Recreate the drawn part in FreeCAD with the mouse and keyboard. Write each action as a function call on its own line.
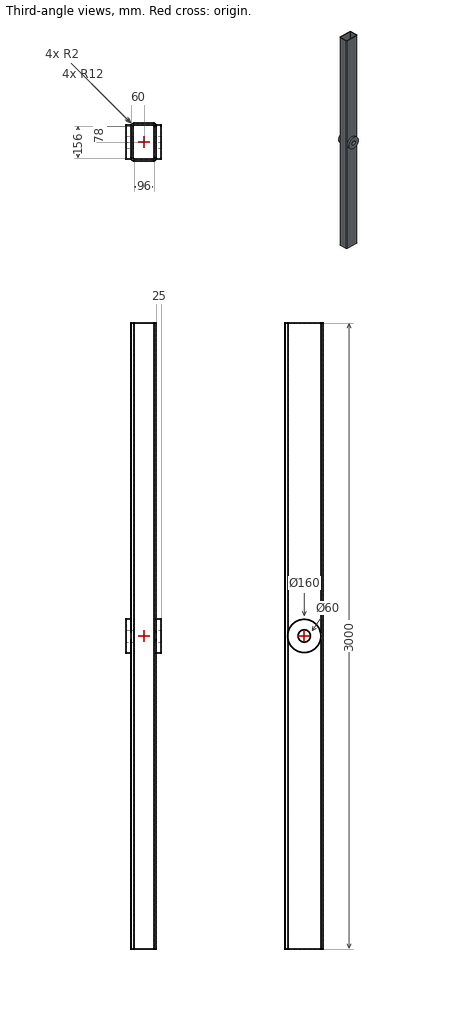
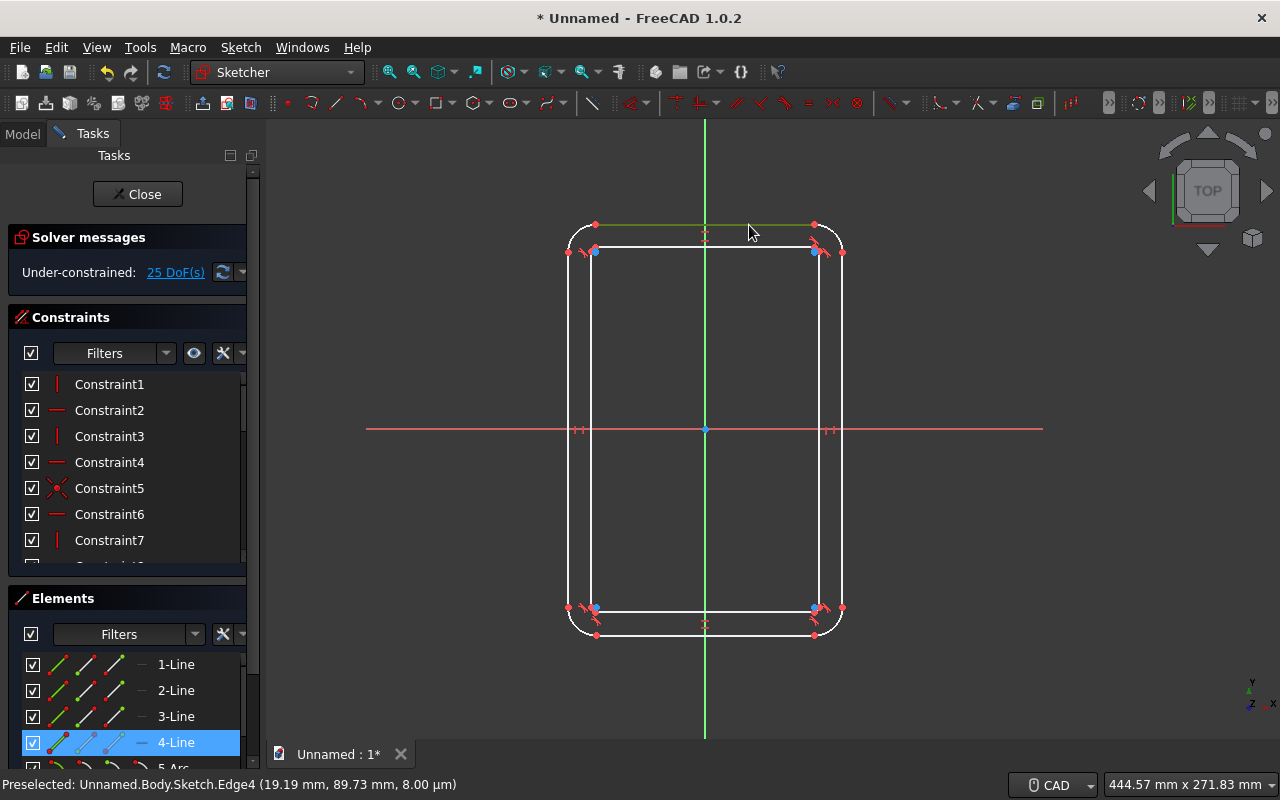
click(583, 228)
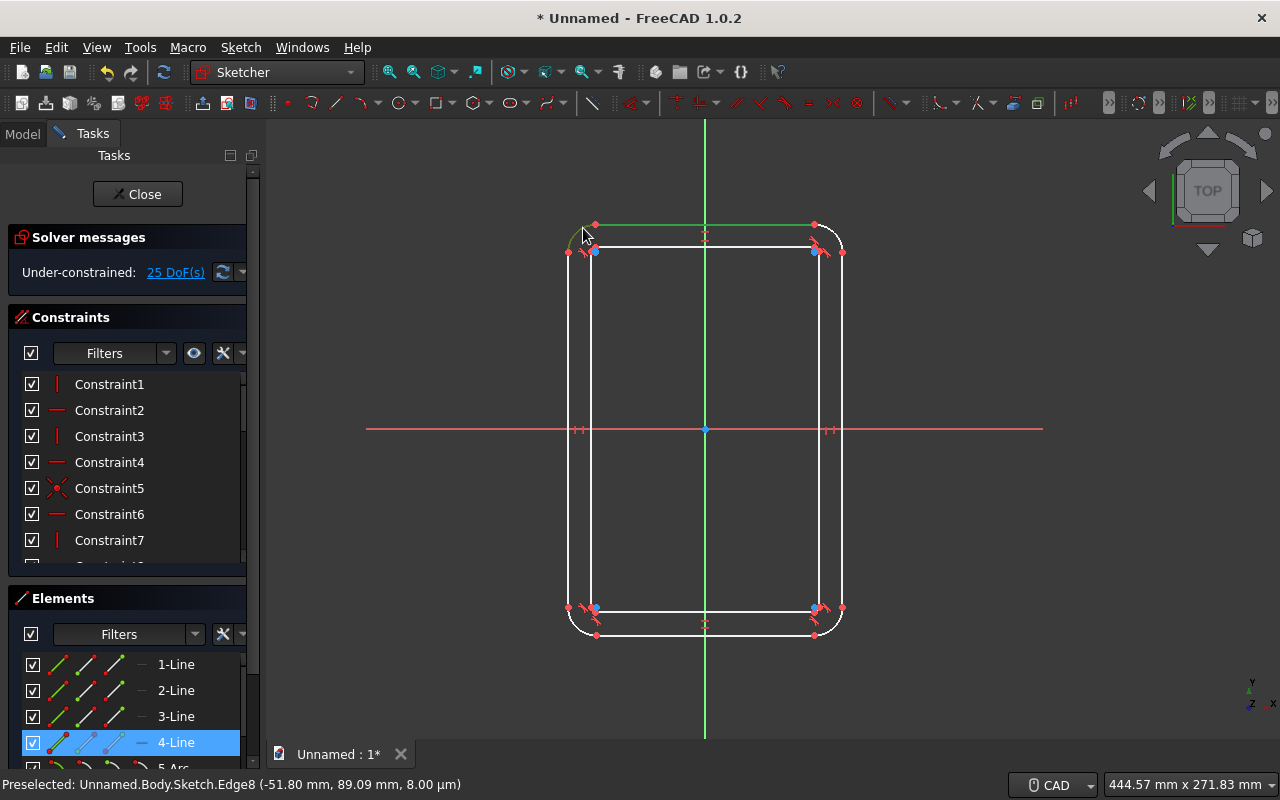
click(786, 104)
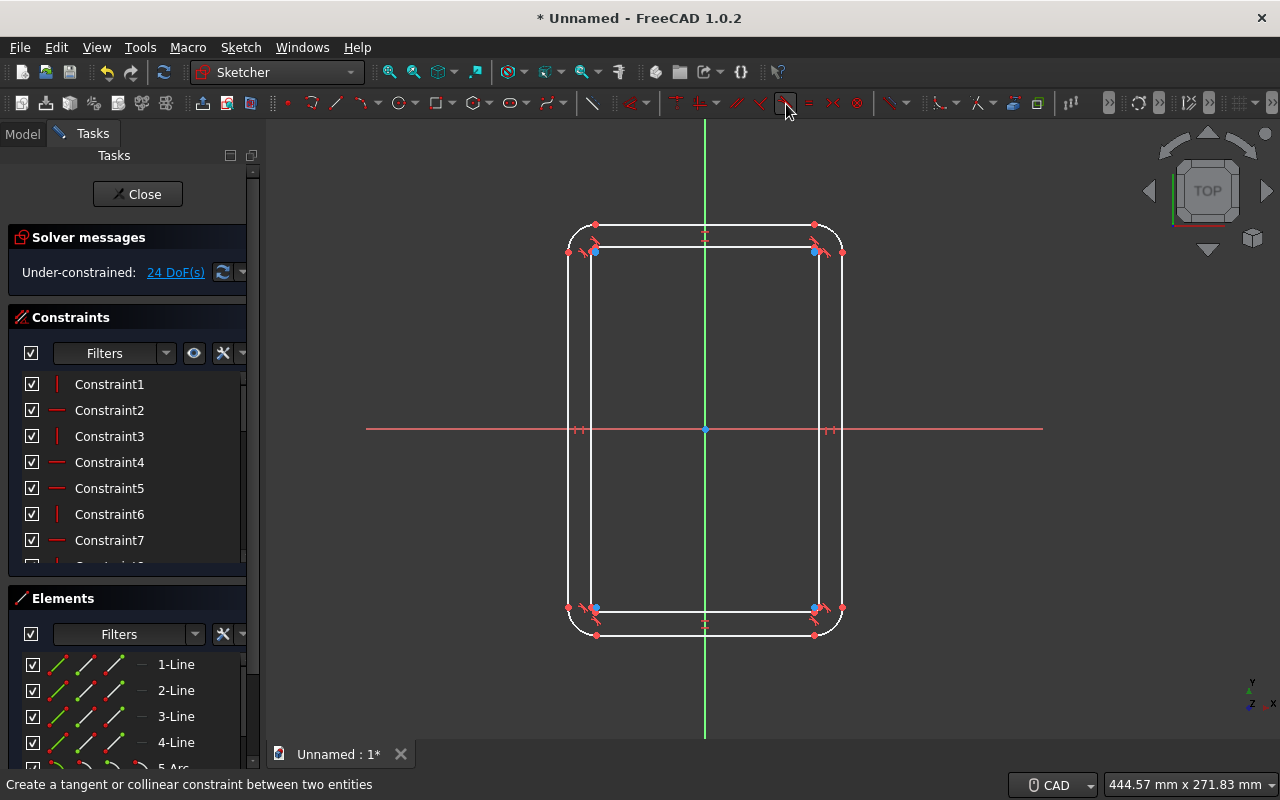
click(661, 247)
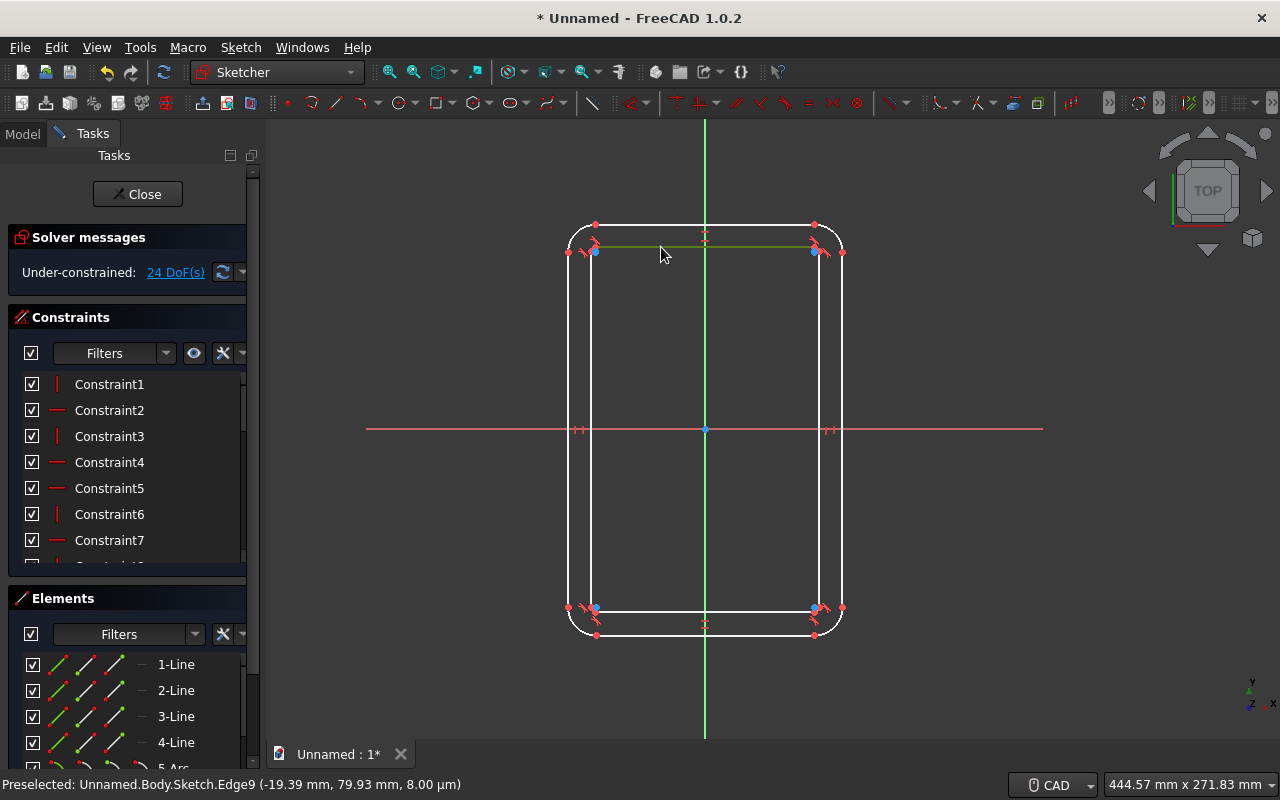
scroll(818, 249, up, 7)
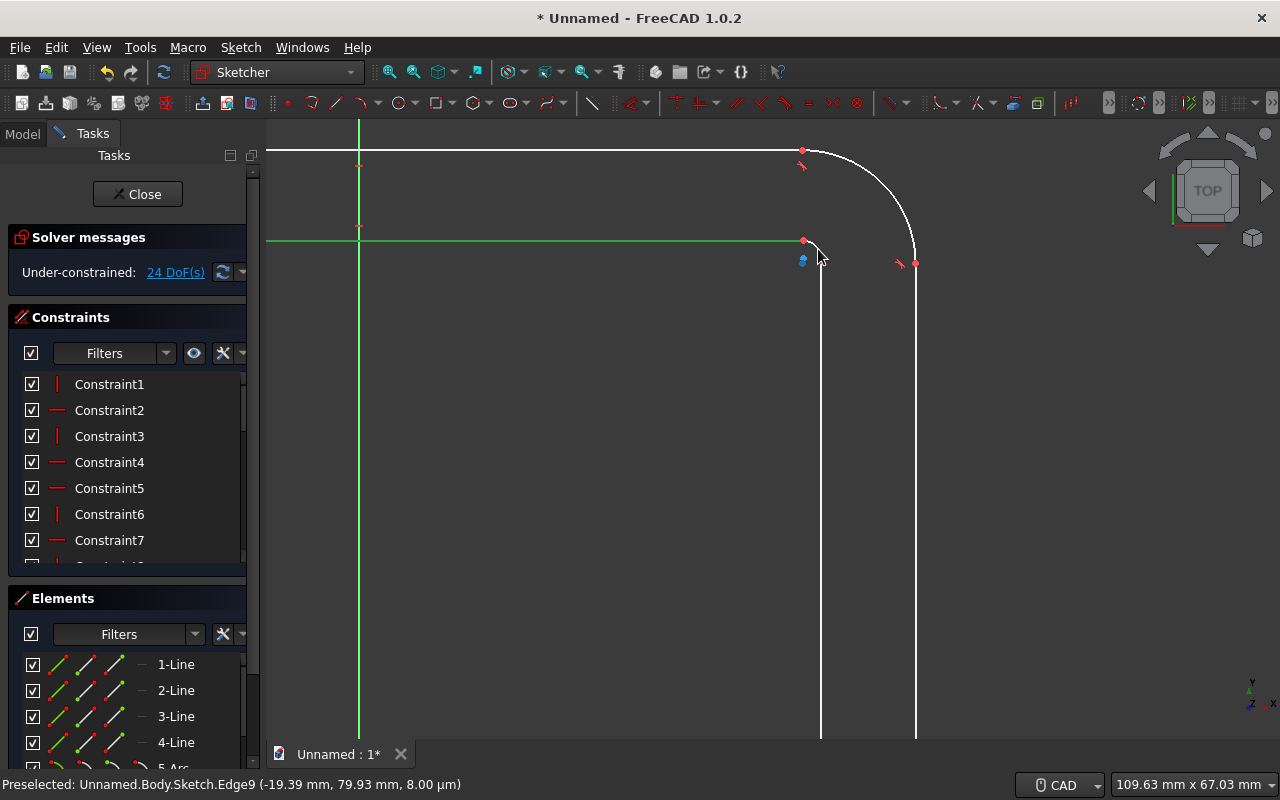
click(816, 247)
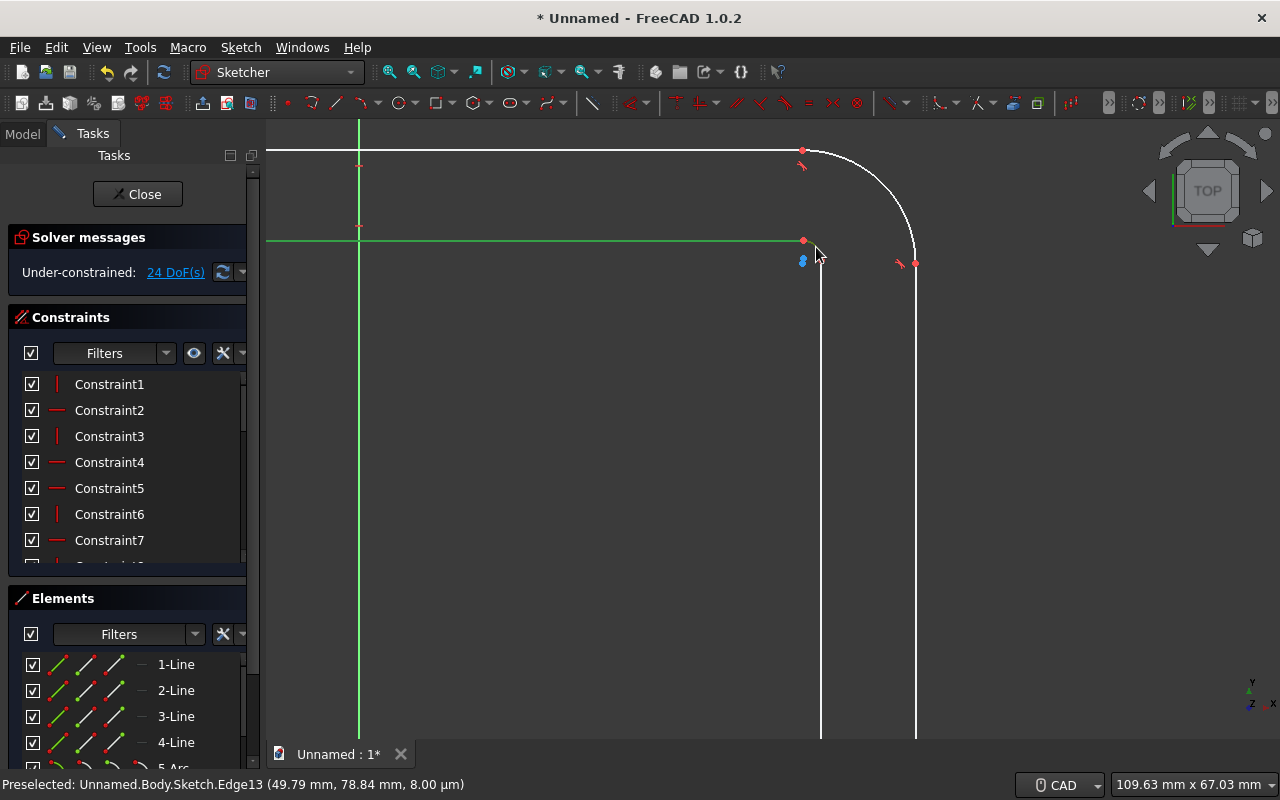
click(786, 104)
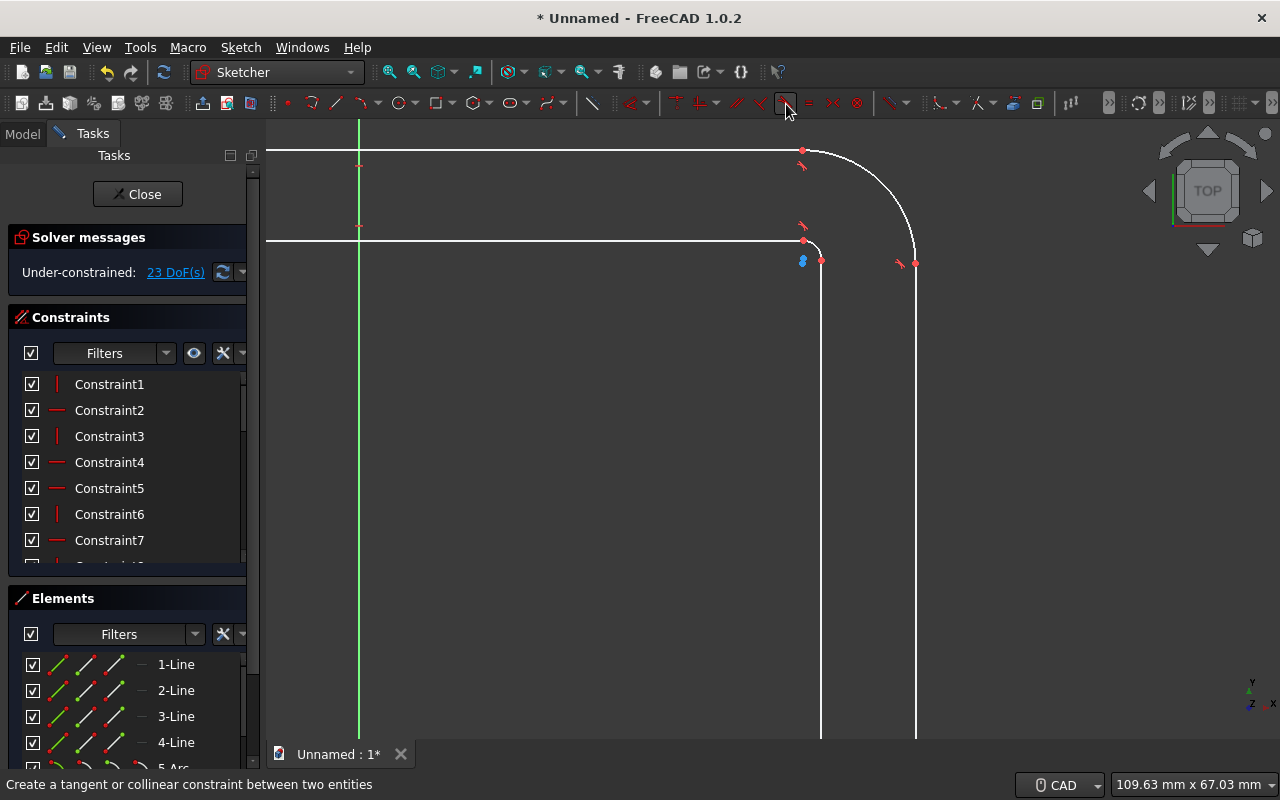
scroll(818, 249, down, 7)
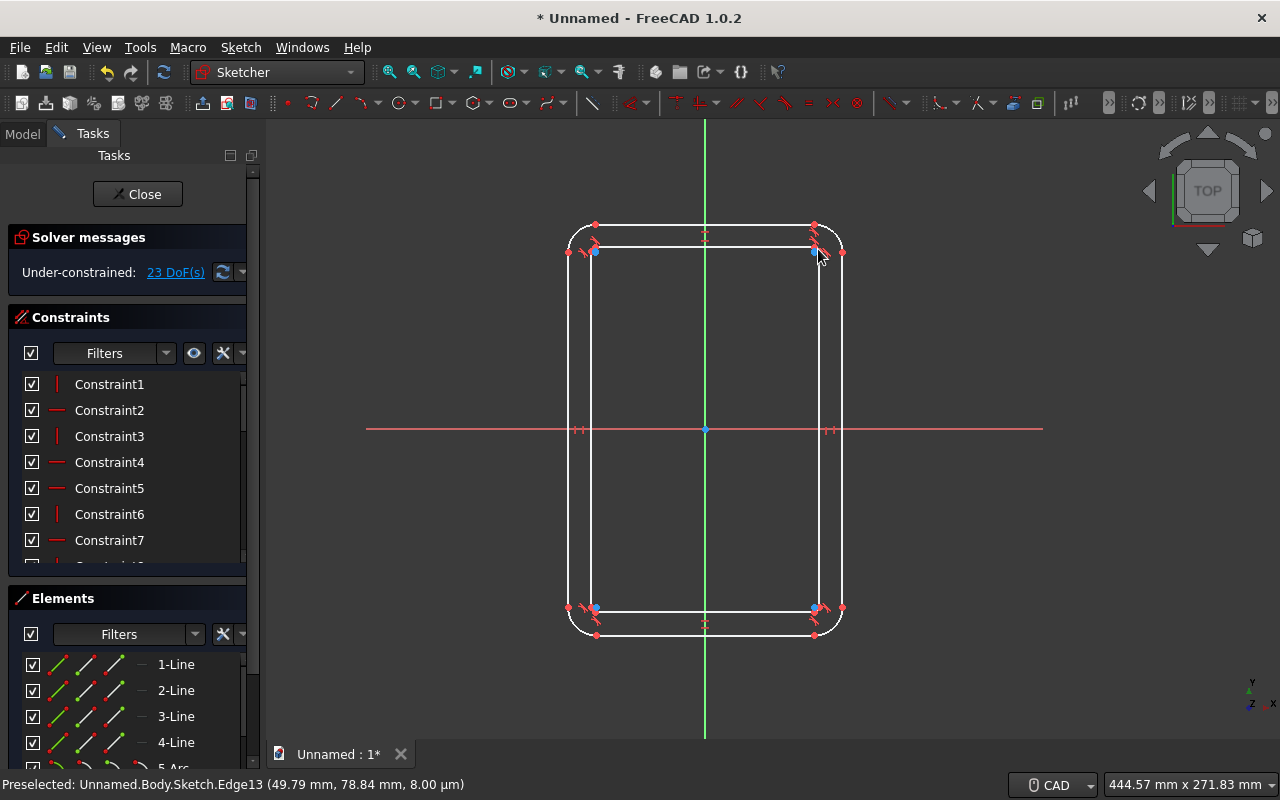
click(749, 247)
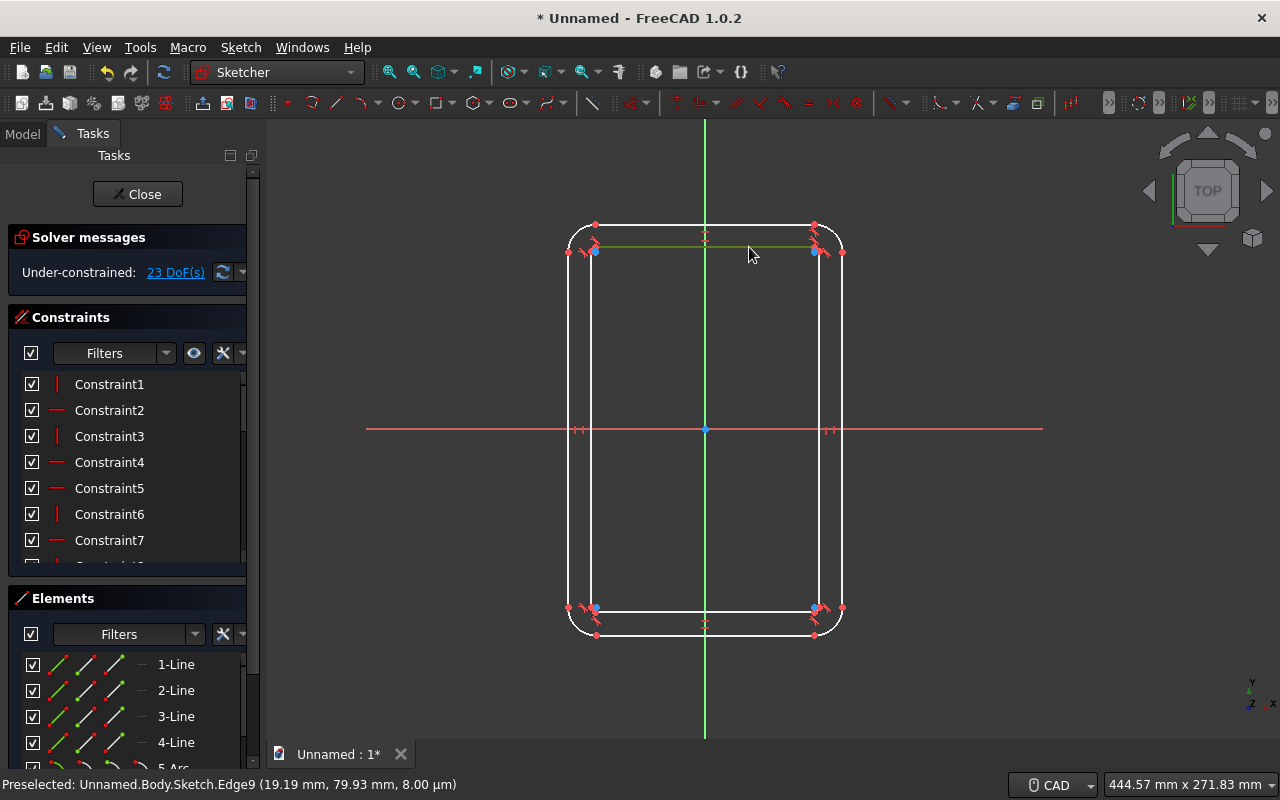
scroll(592, 248, up, 7)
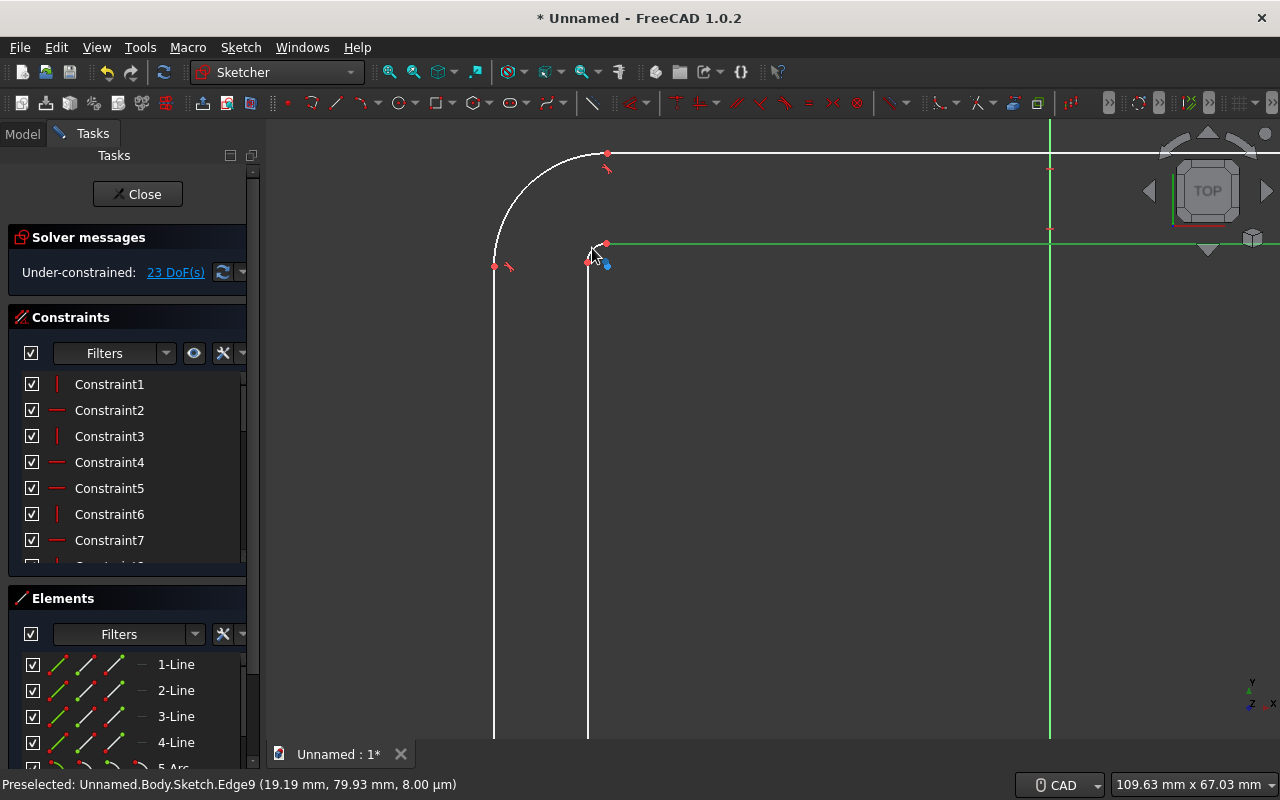
click(593, 249)